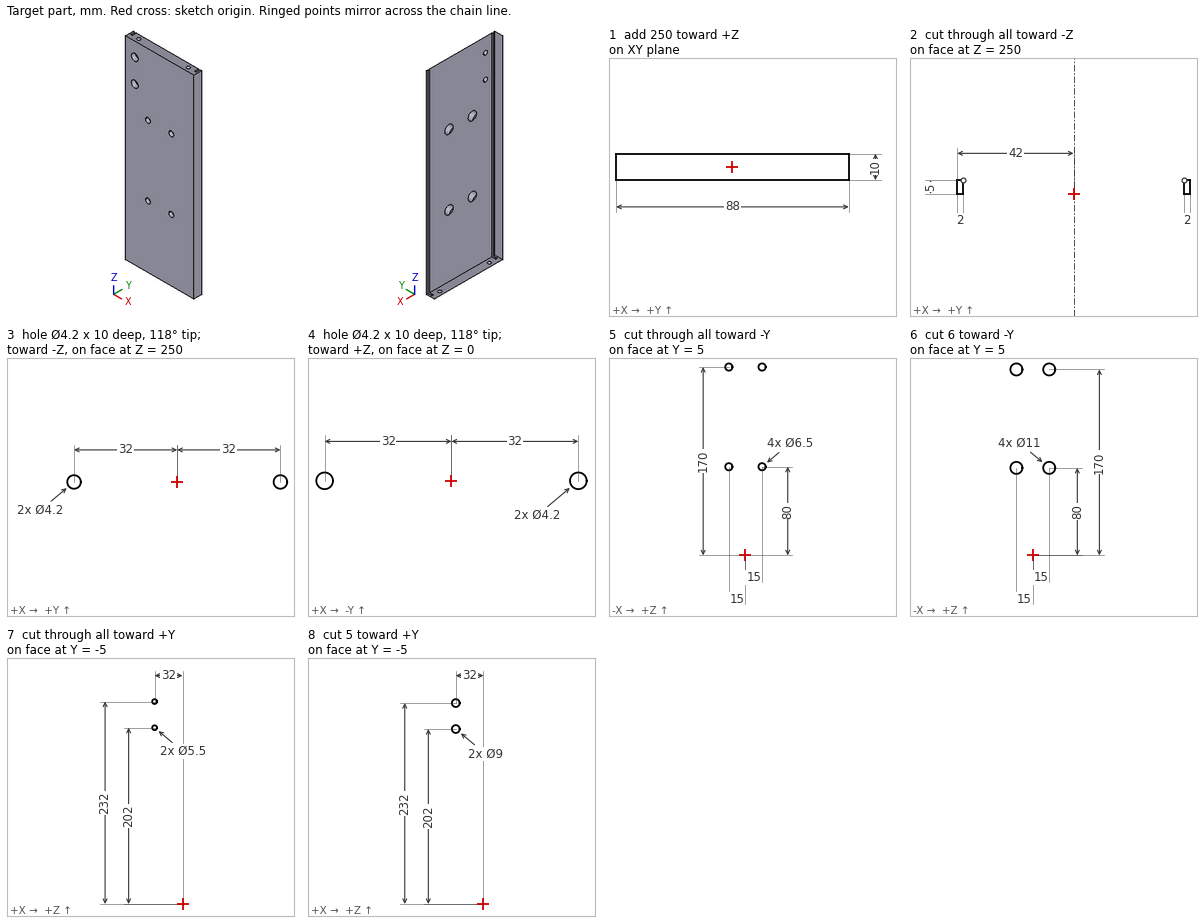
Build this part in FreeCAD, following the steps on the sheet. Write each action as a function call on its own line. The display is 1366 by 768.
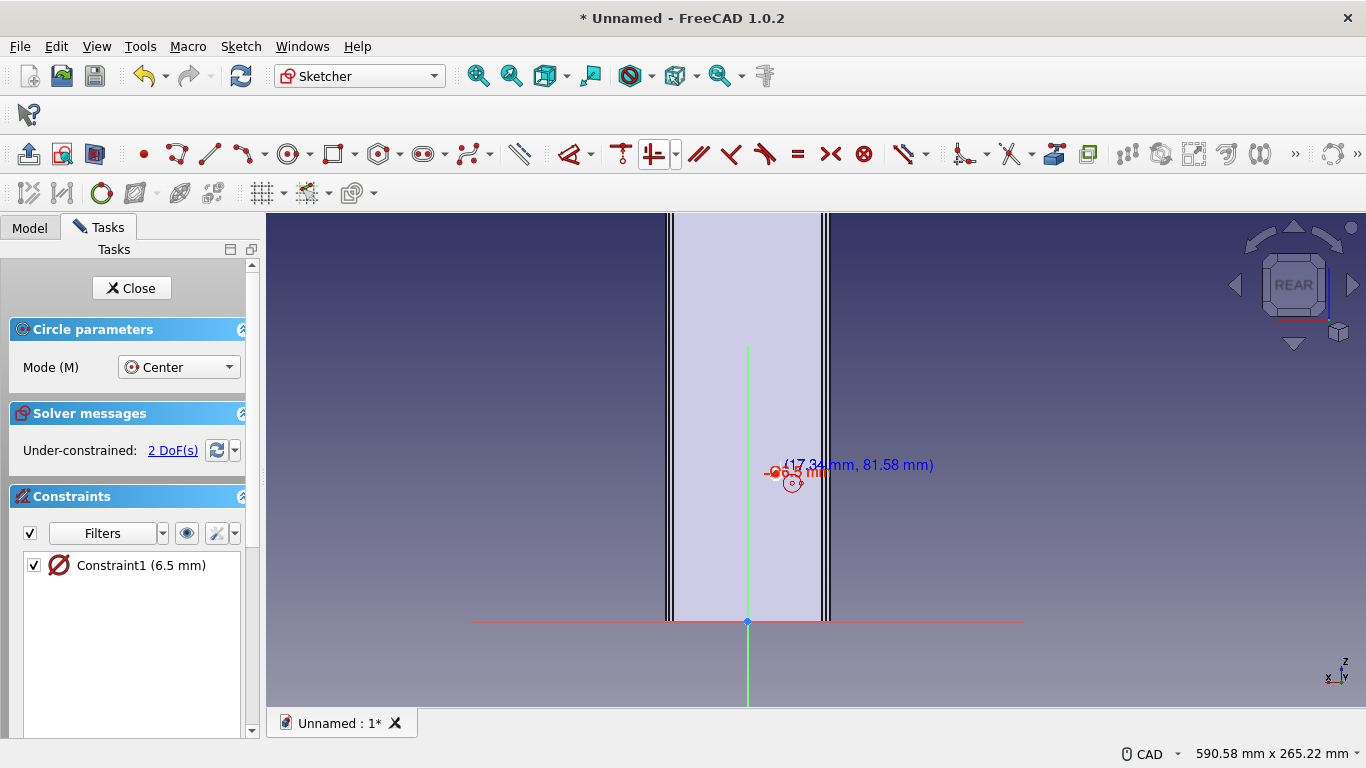
scroll(720, 473, up, 7)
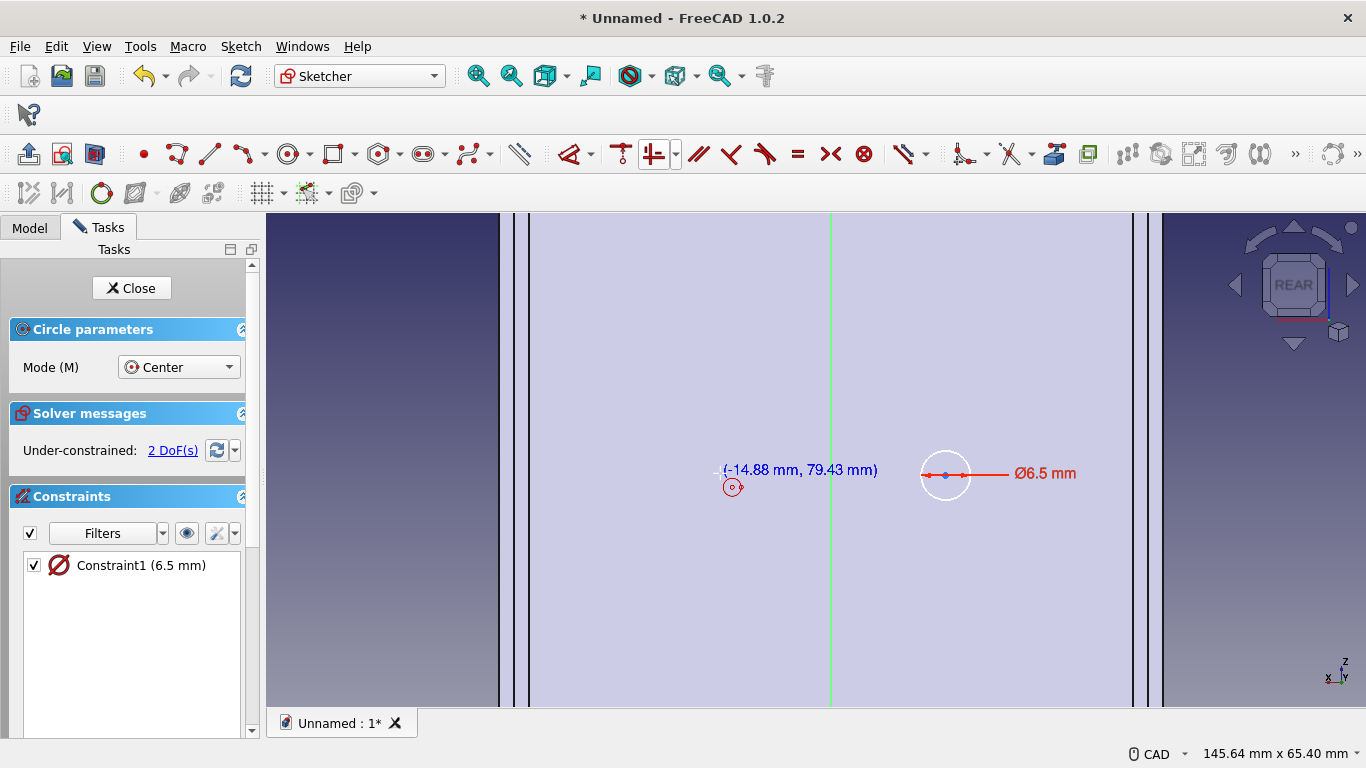
scroll(720, 473, down, 7)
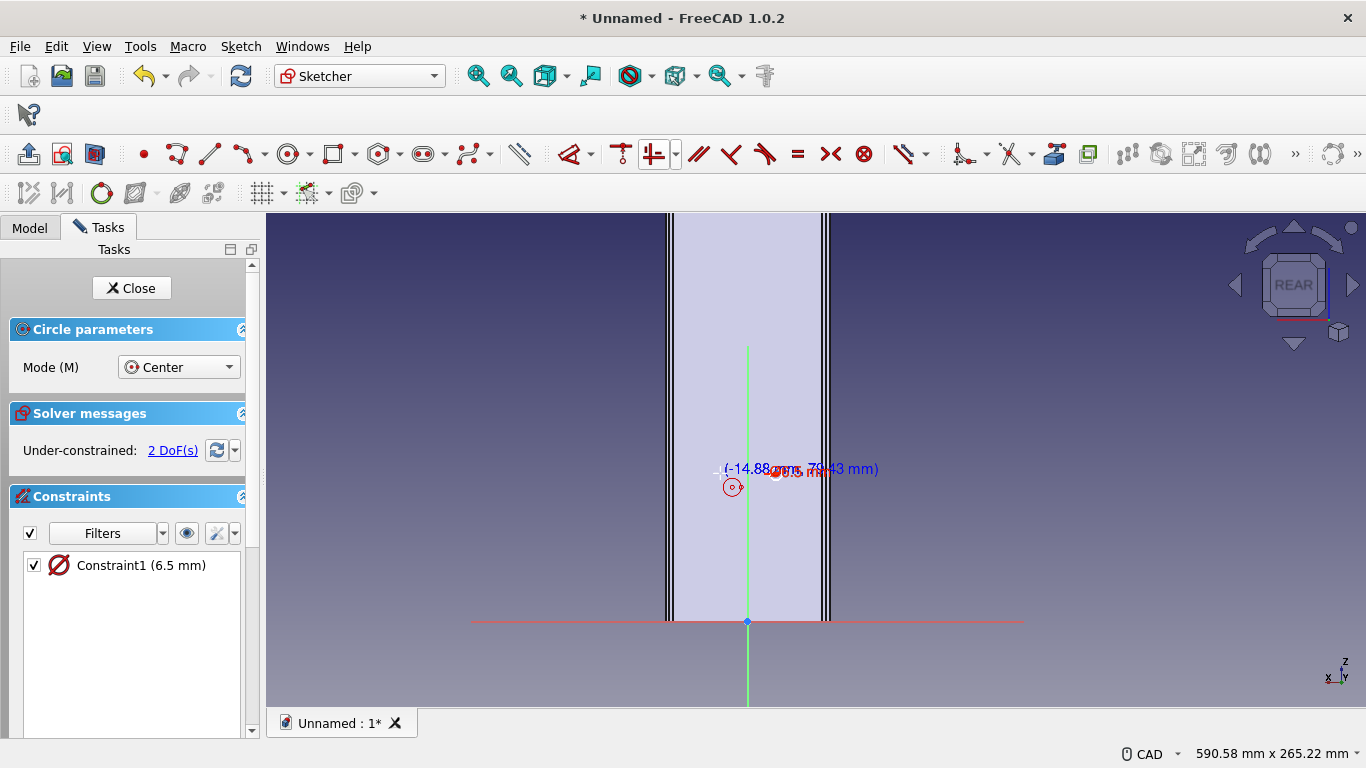
click(720, 473)
move(724, 469)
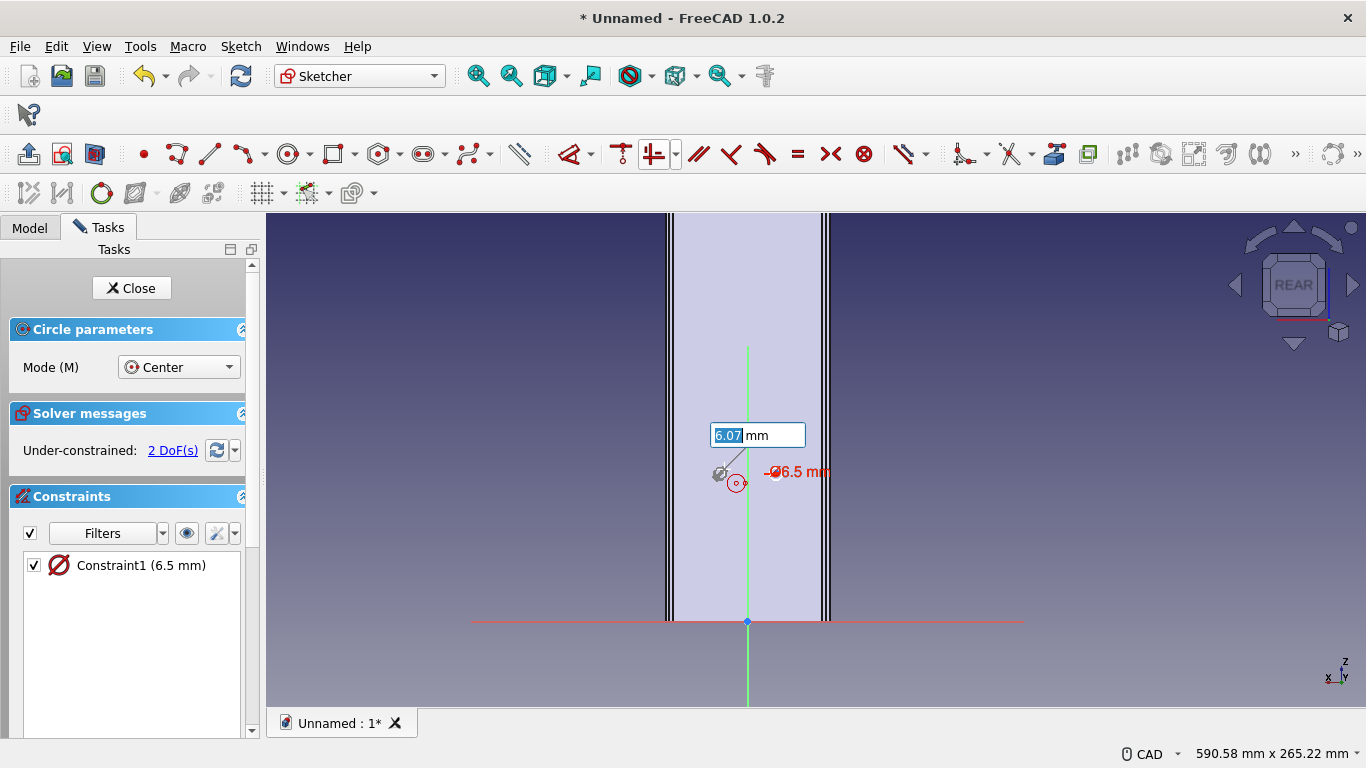
text(6.5)
key(Return)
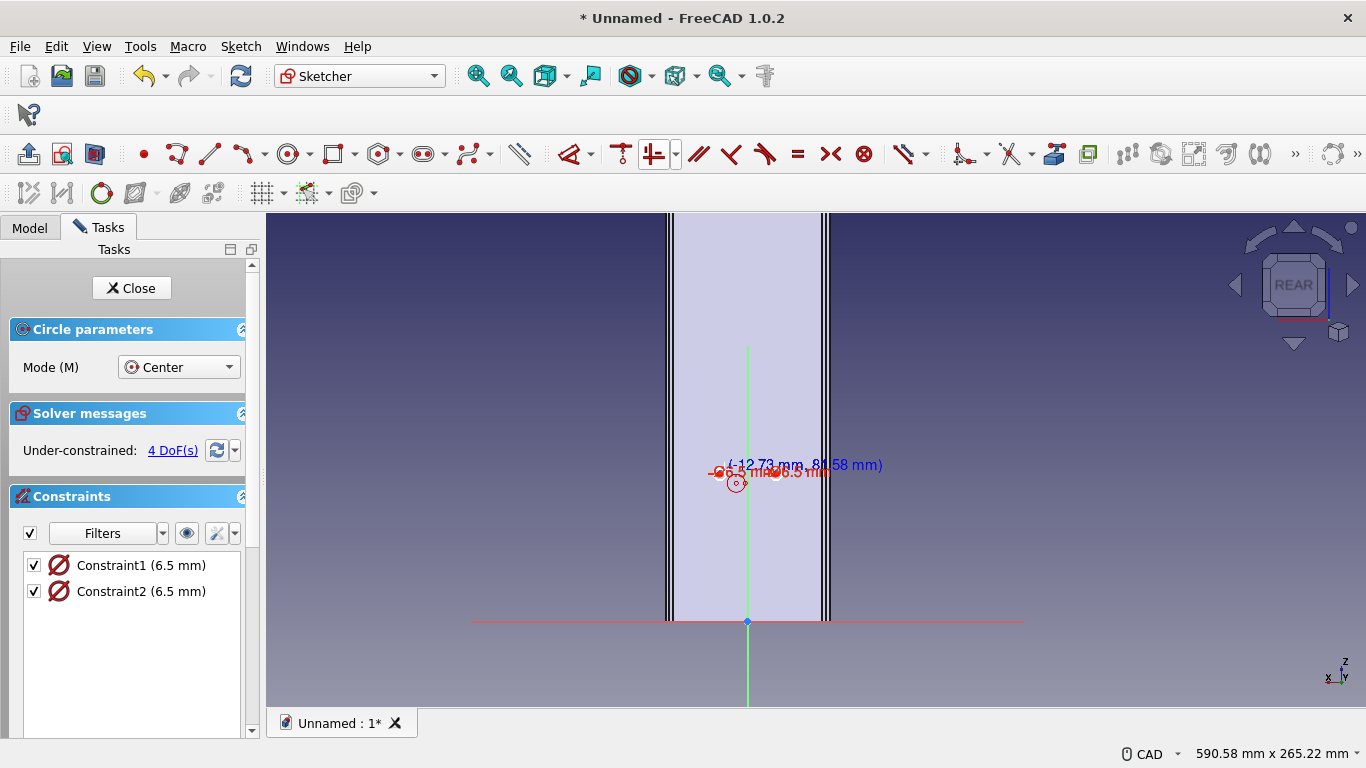
scroll(720, 305, up, 7)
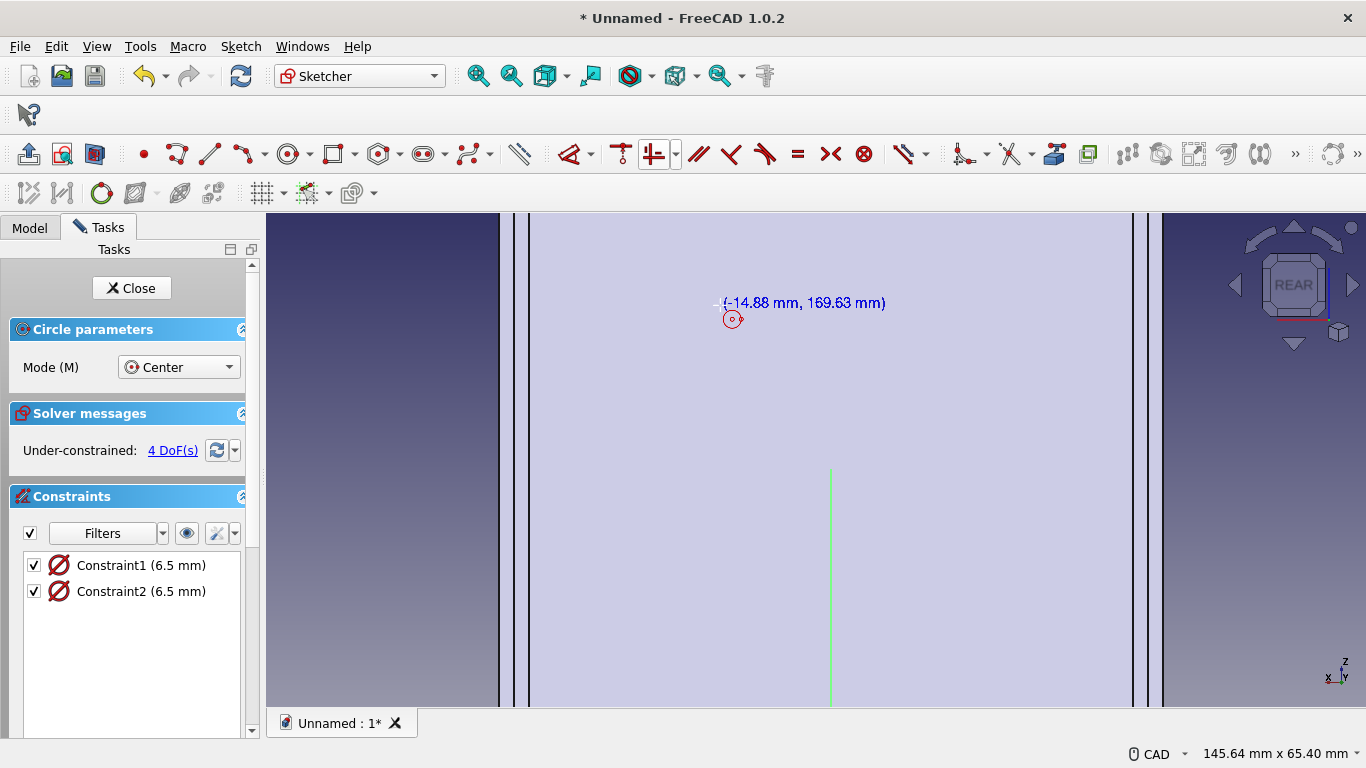
scroll(720, 304, down, 7)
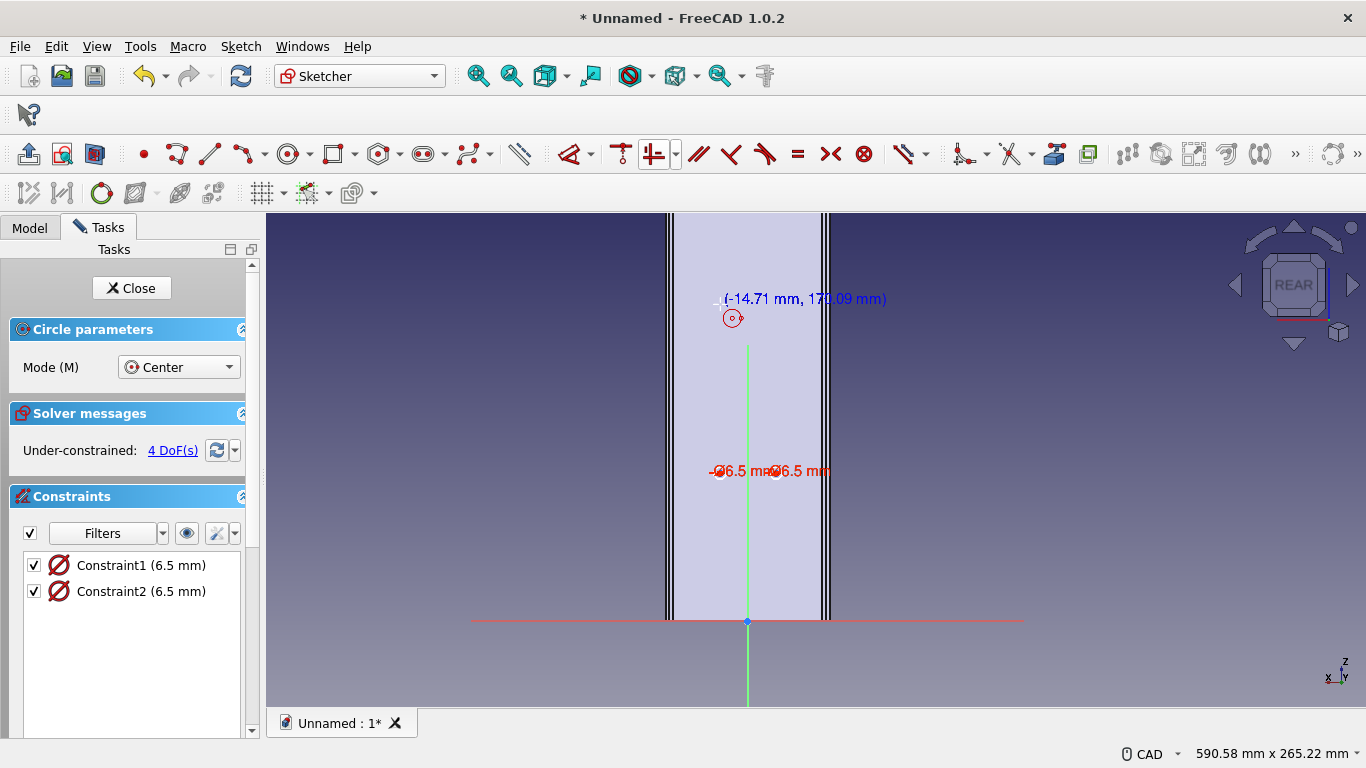
click(720, 305)
move(724, 300)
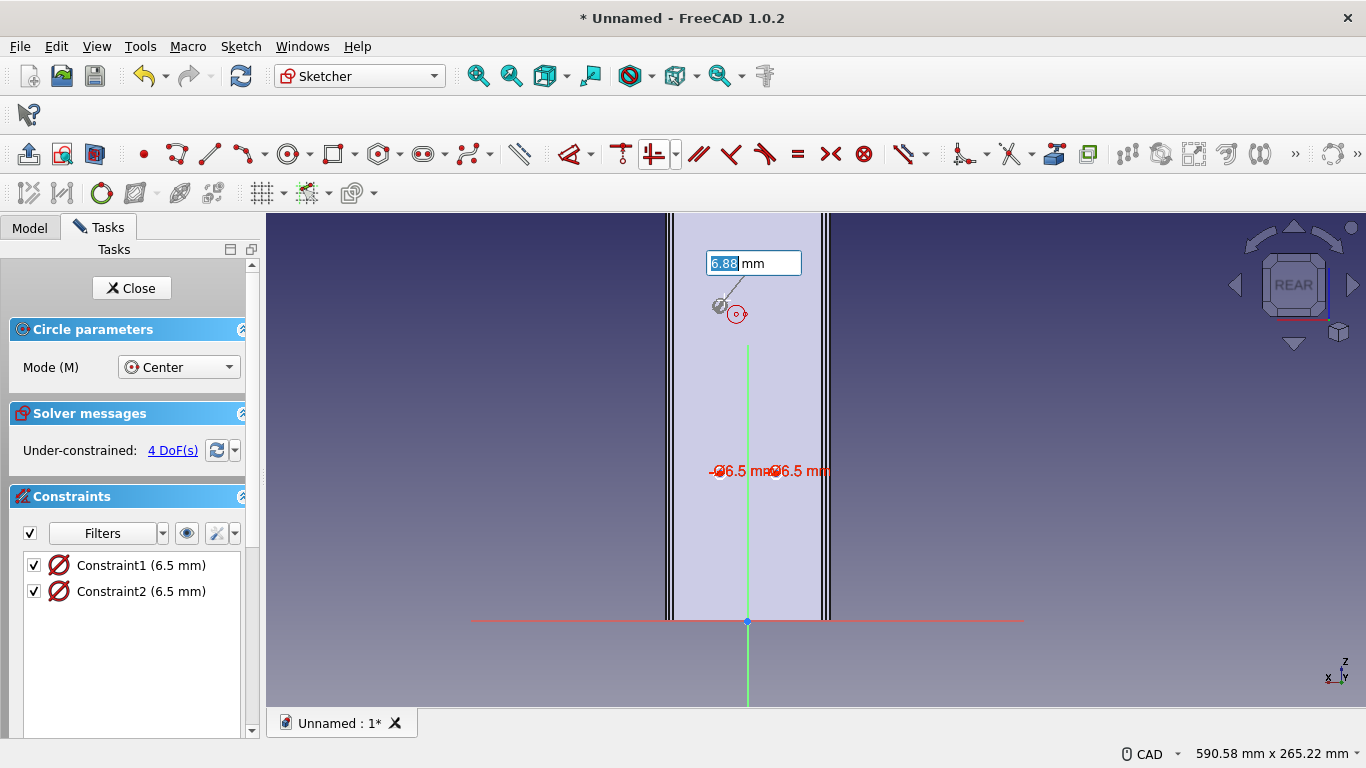
text(6.5)
key(Return)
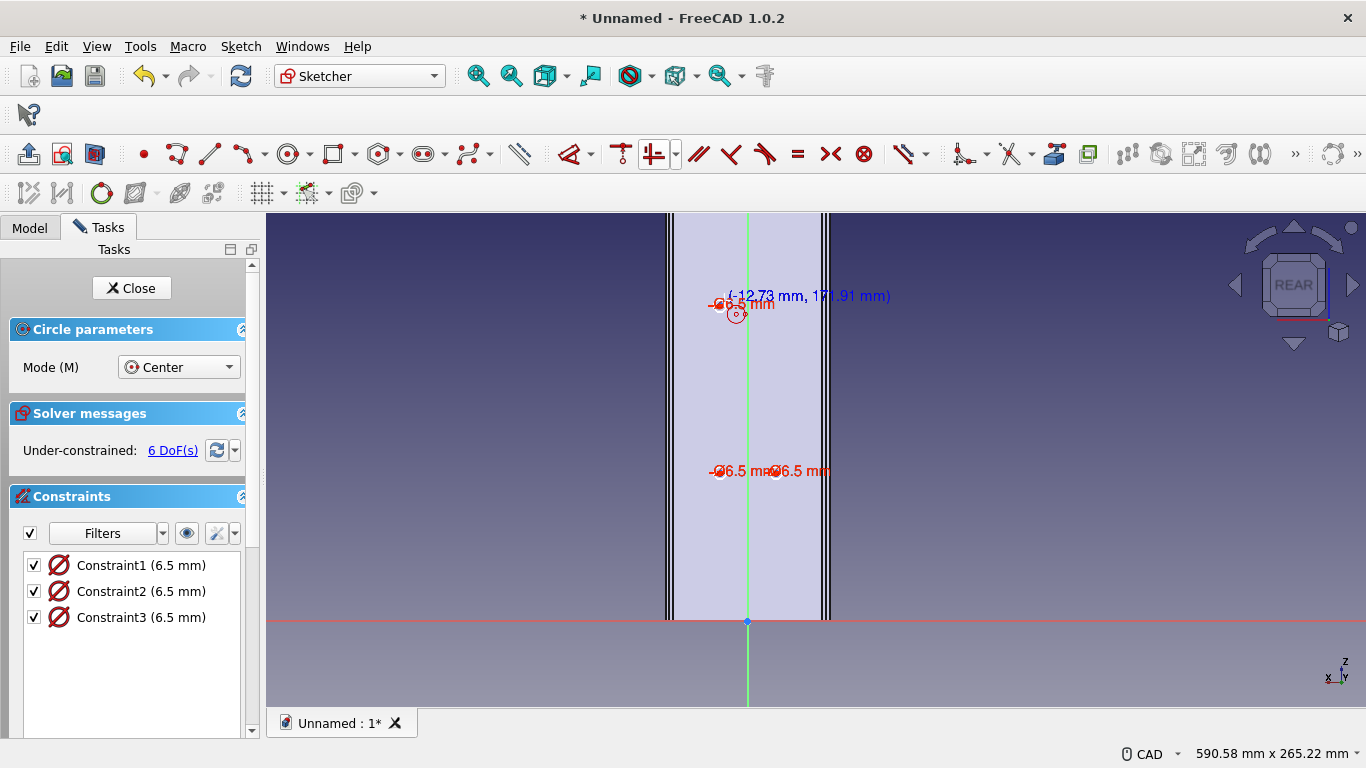
scroll(776, 305, up, 7)